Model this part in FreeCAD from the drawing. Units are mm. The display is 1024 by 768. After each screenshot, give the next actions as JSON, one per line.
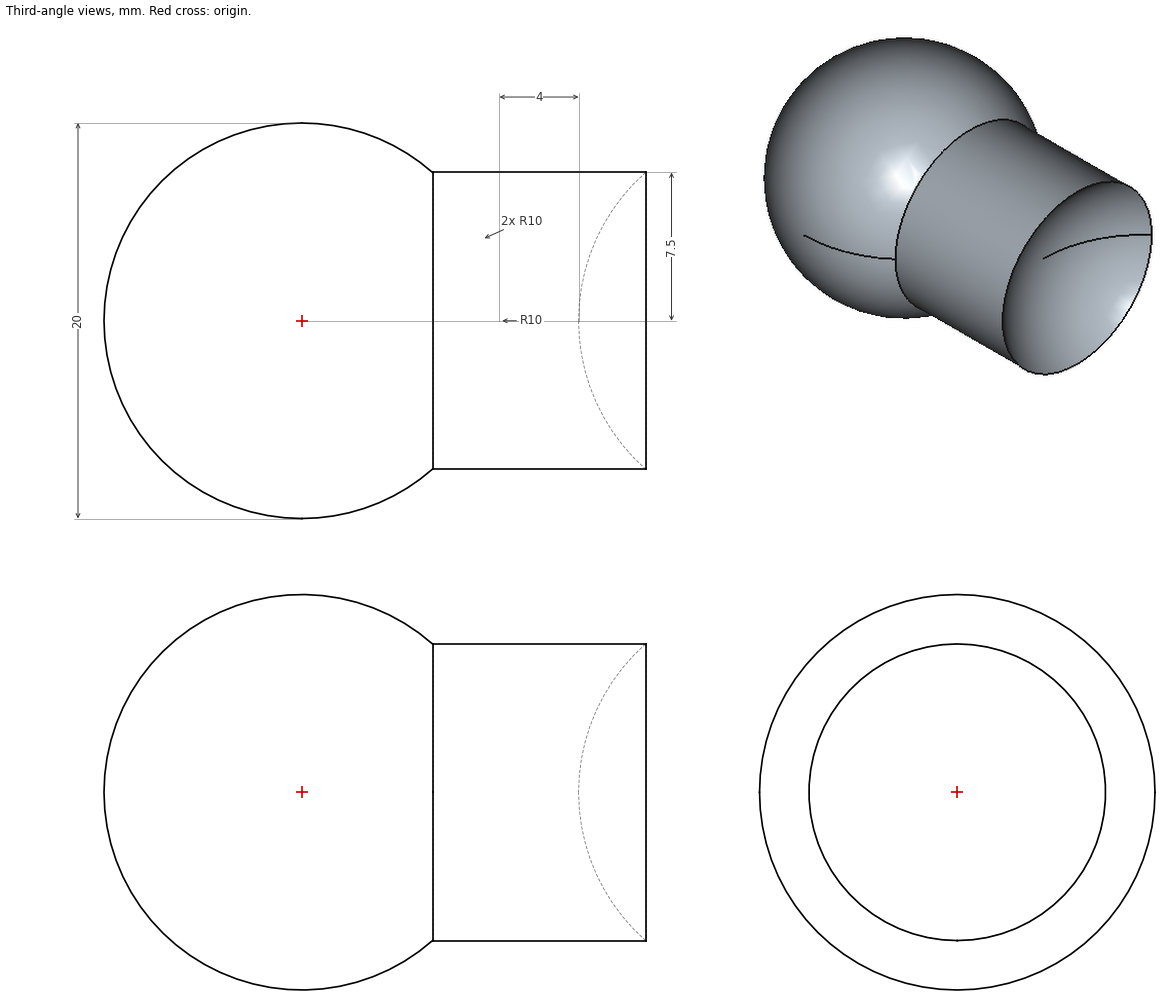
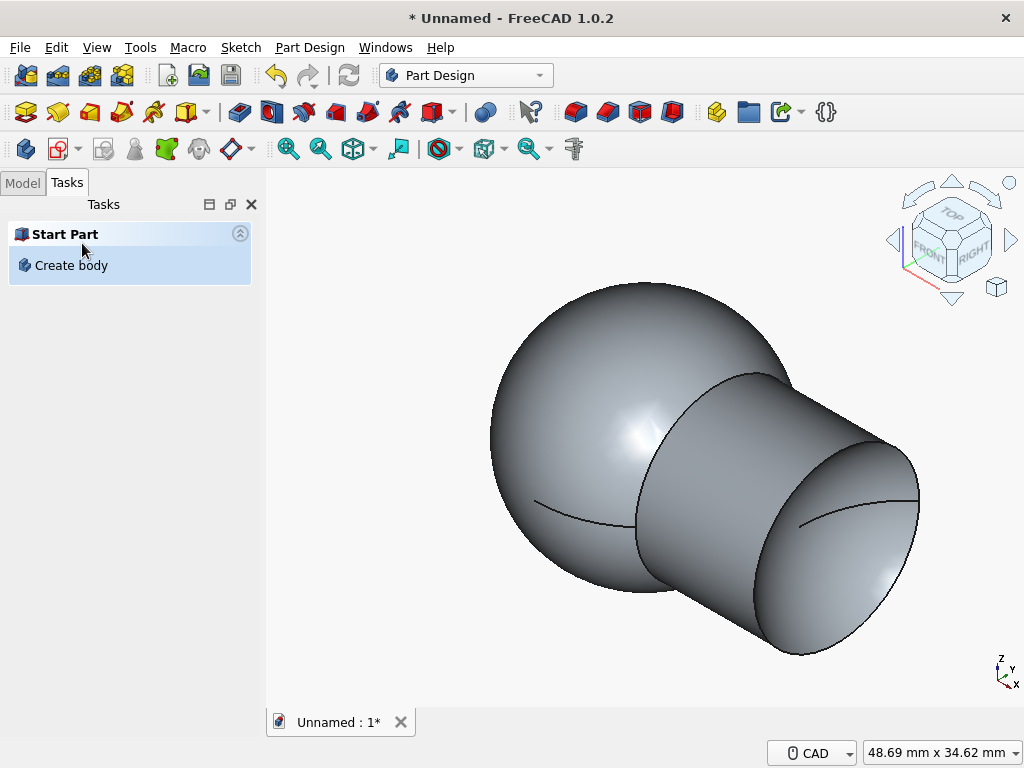
{"action": "key", "text": "v f"}